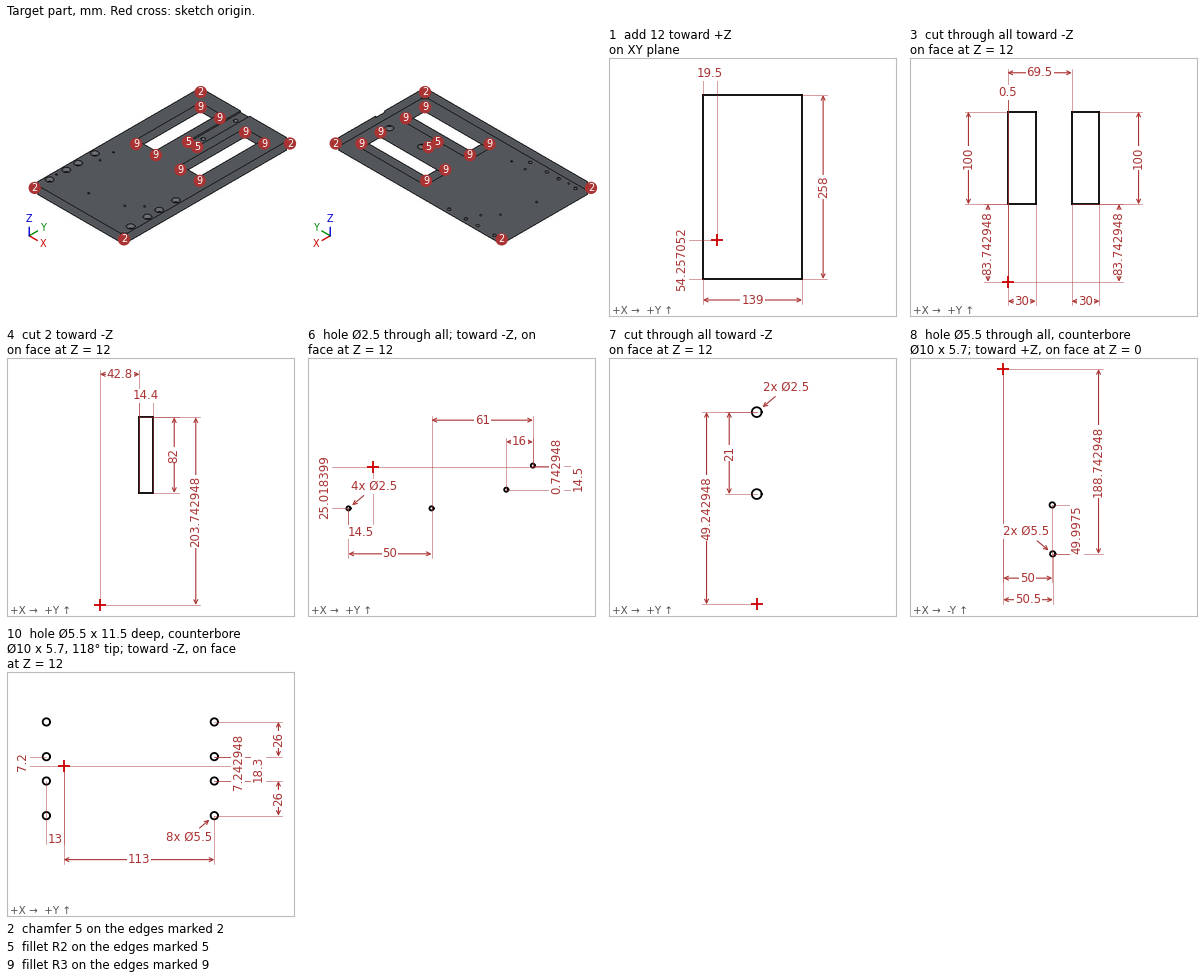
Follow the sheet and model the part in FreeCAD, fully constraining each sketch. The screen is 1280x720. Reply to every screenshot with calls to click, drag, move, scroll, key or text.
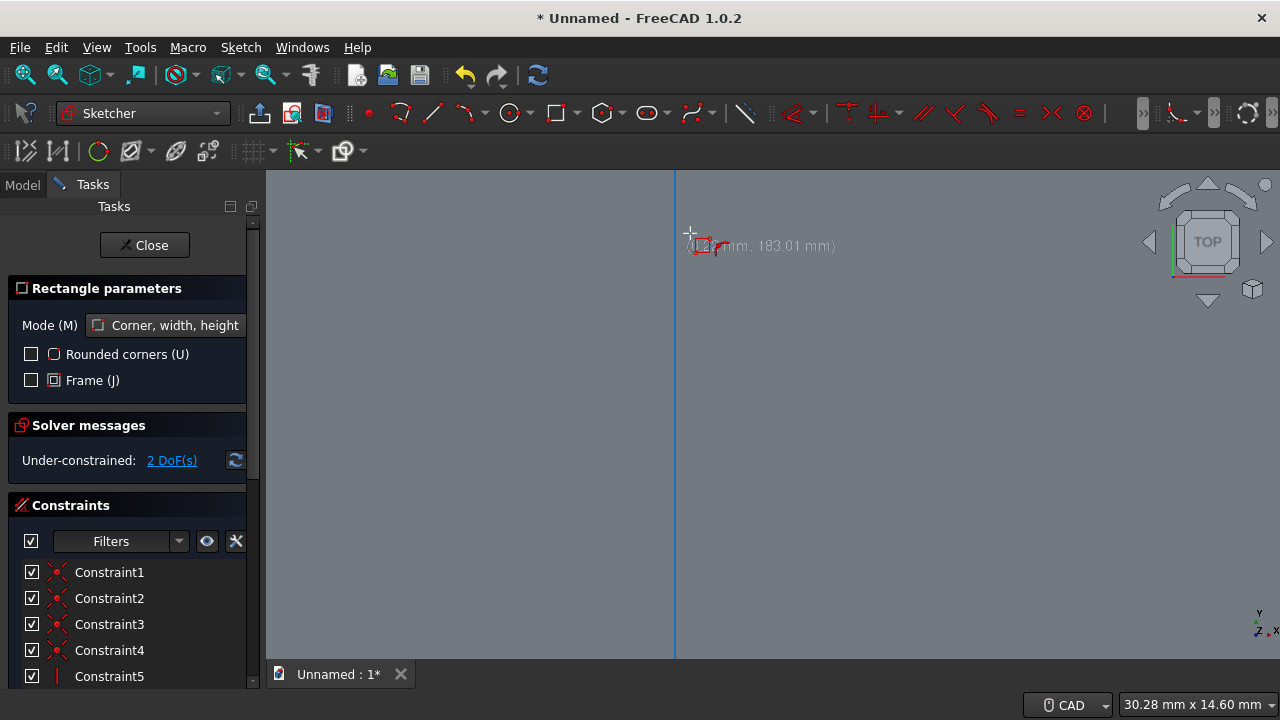
click(692, 226)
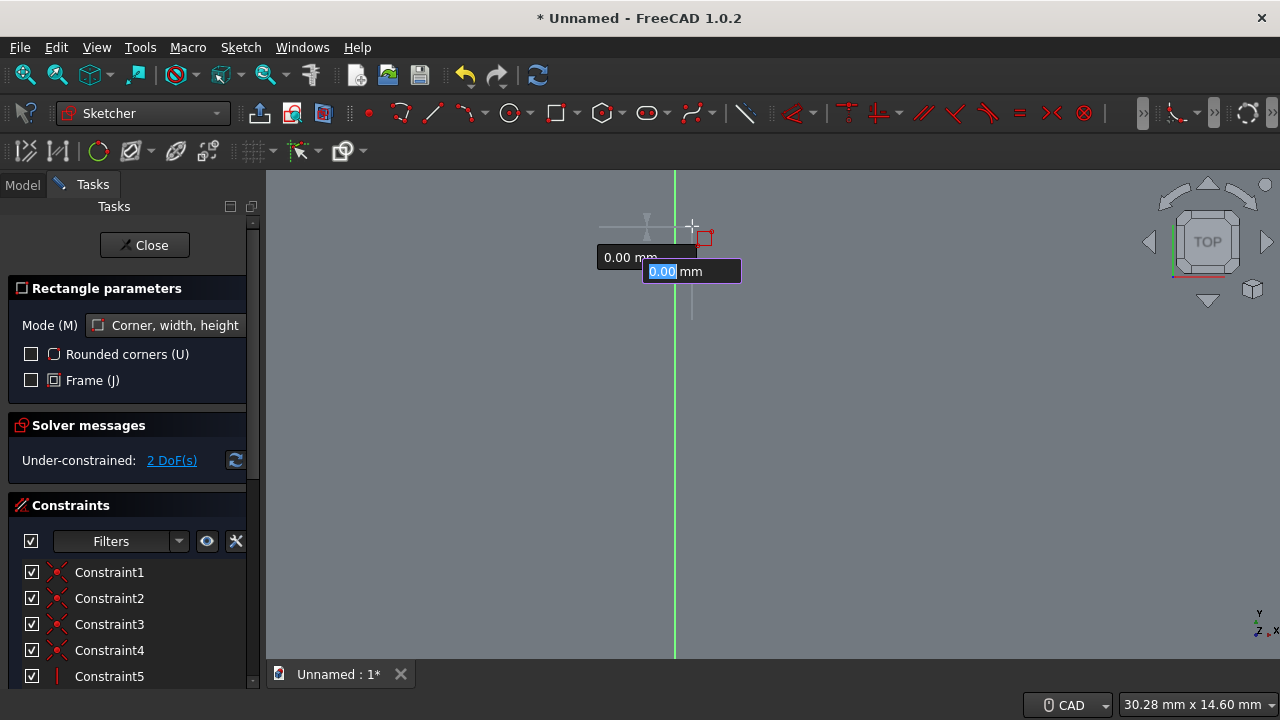
scroll(619, 263, down, 15)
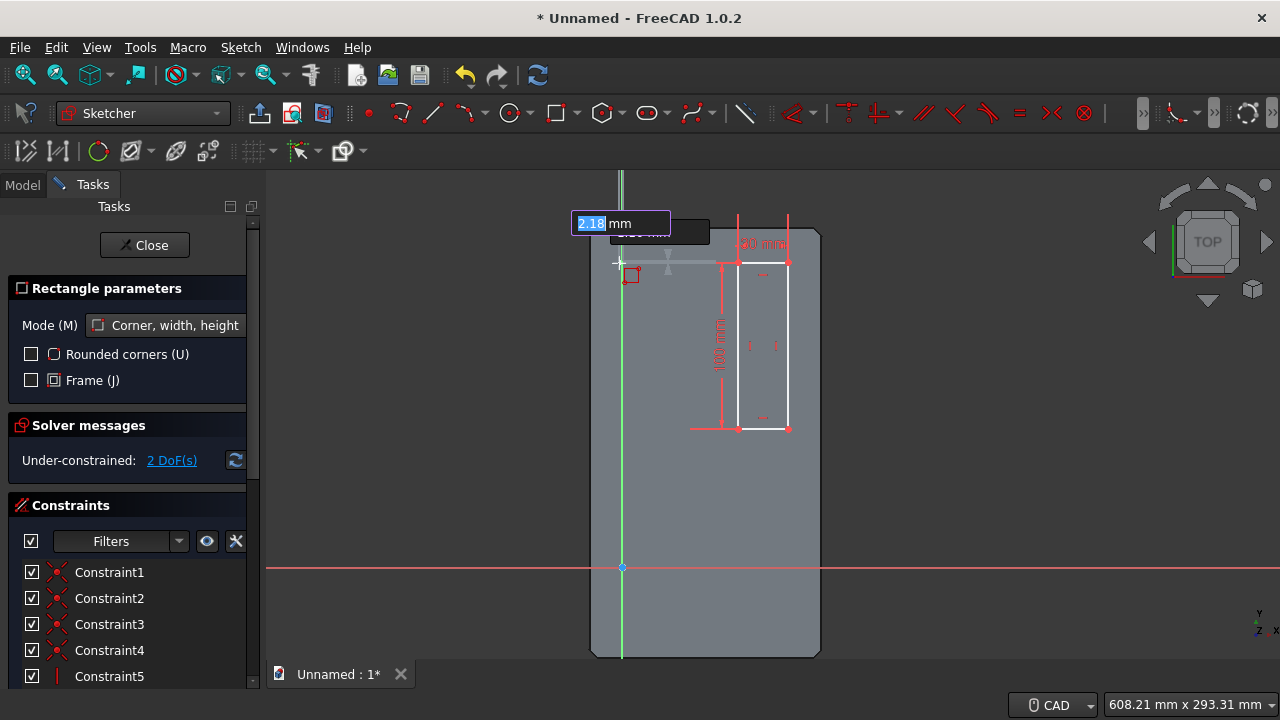
click(673, 428)
key(Escape)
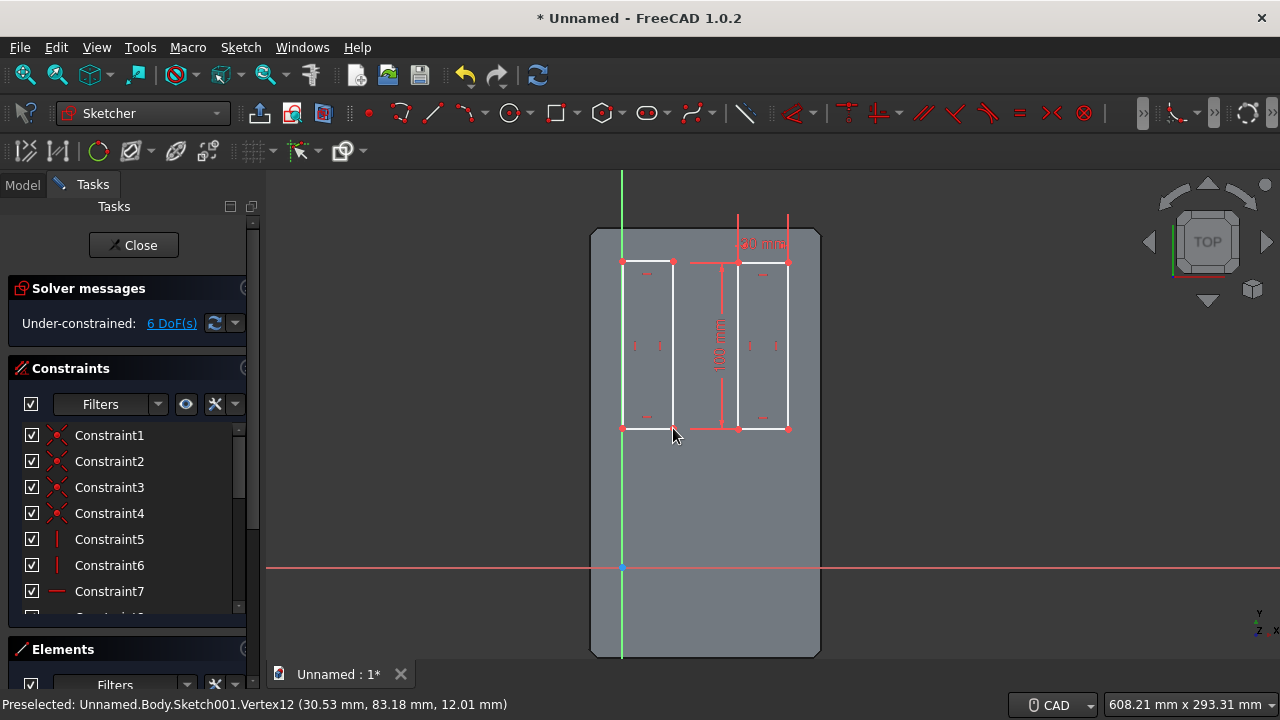
key(d)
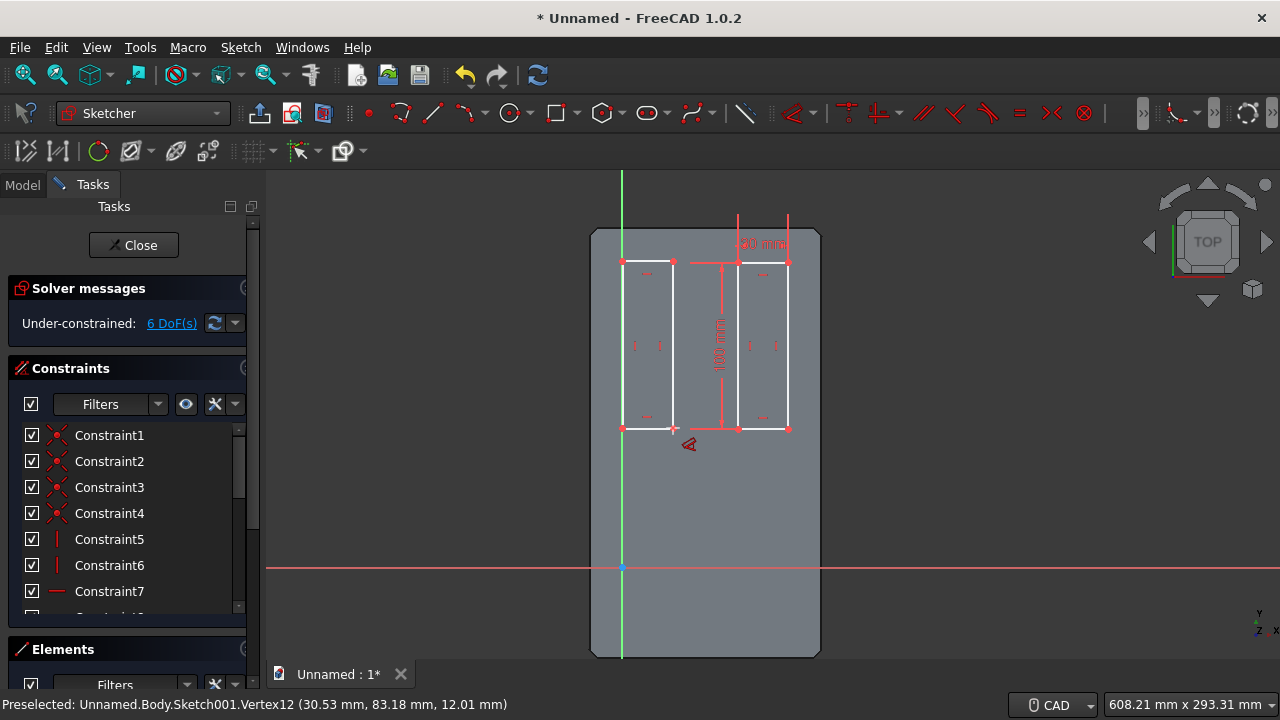
click(638, 429)
click(648, 463)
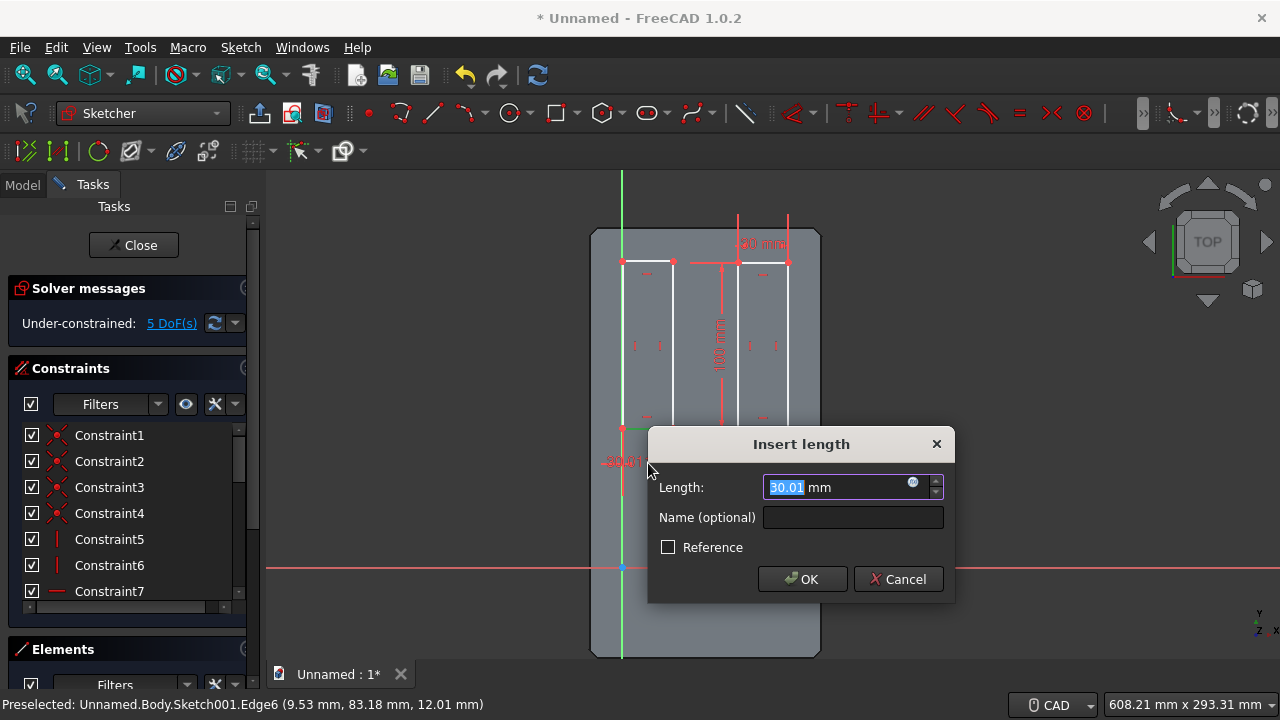
text(30)
key(Return)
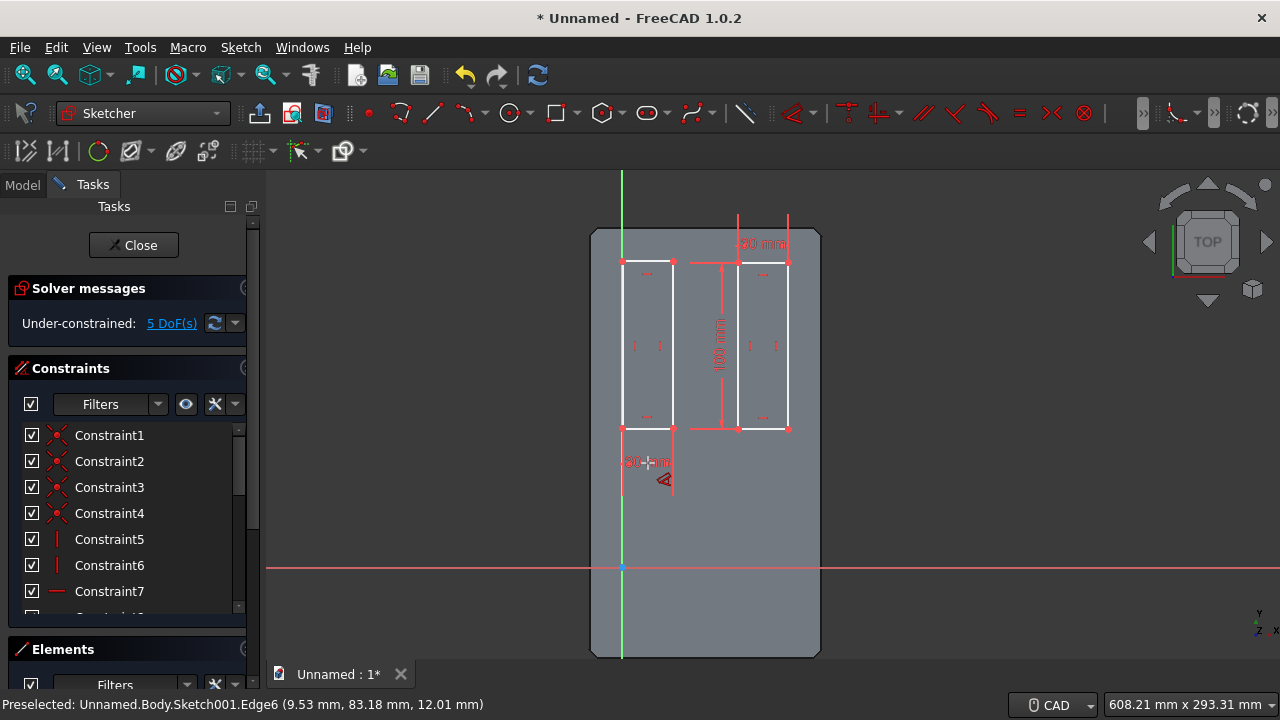
click(623, 312)
click(589, 345)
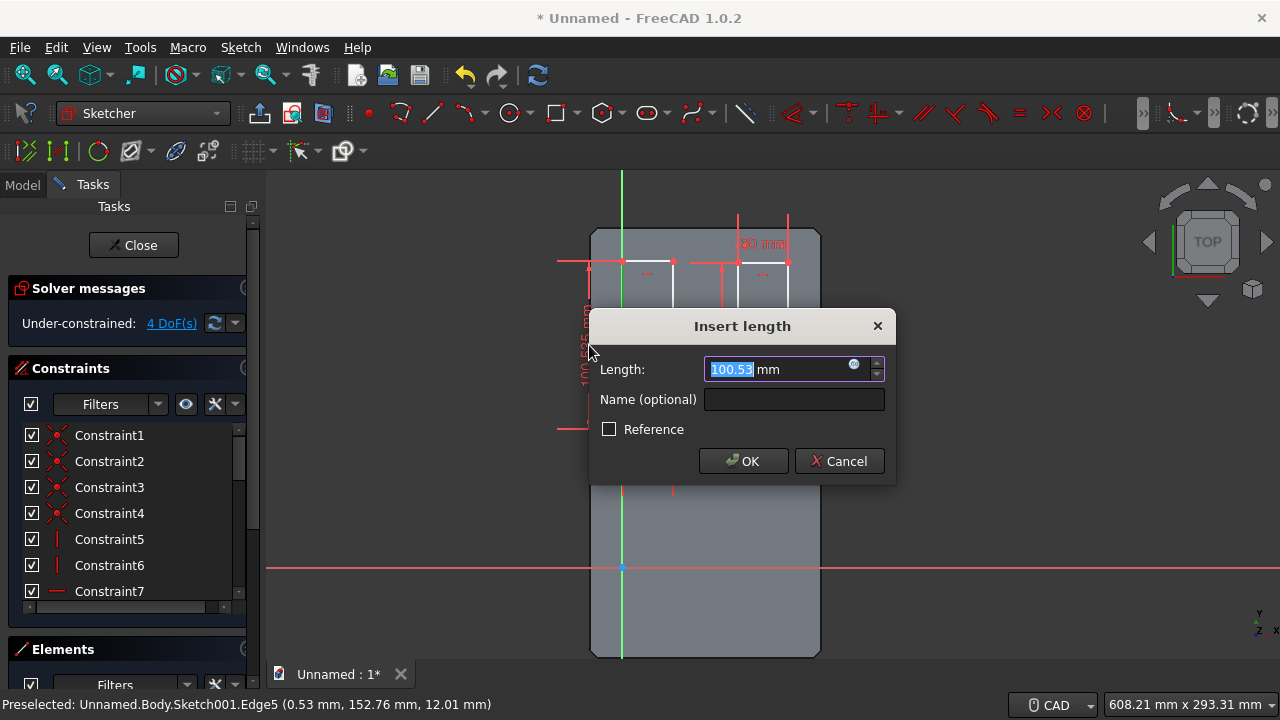
text(100)
key(Return)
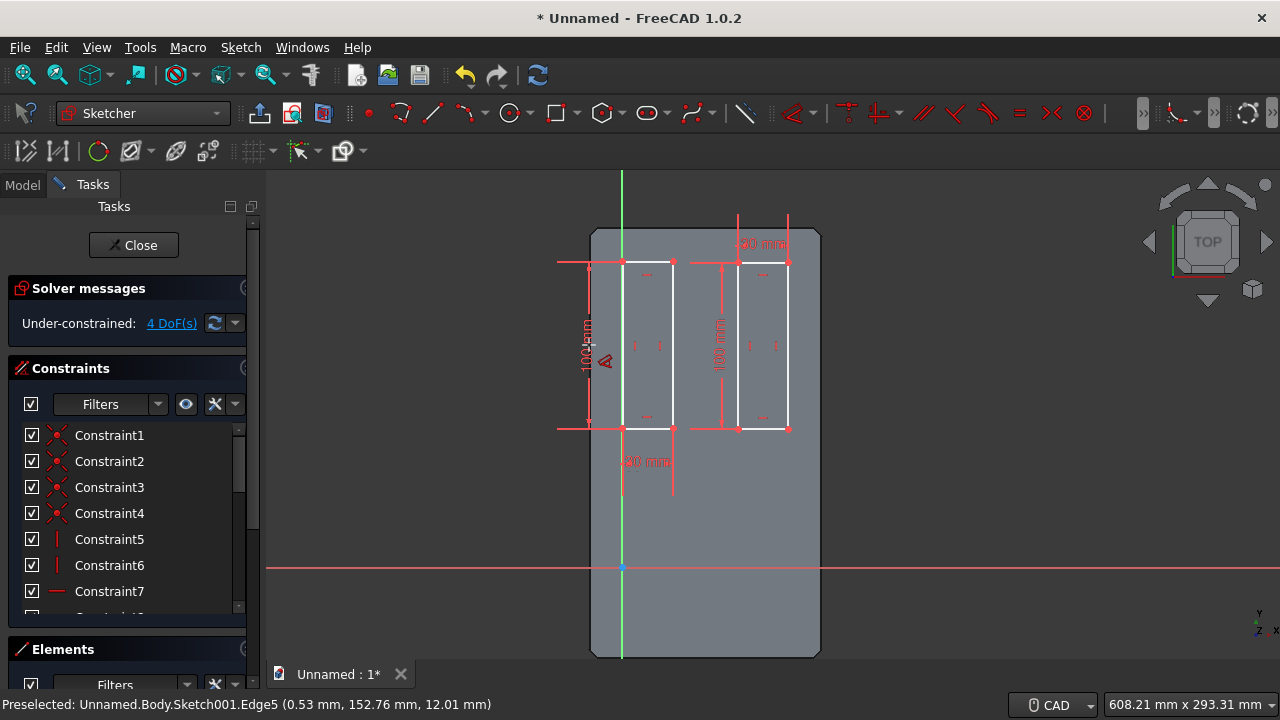
scroll(623, 262, up, 20)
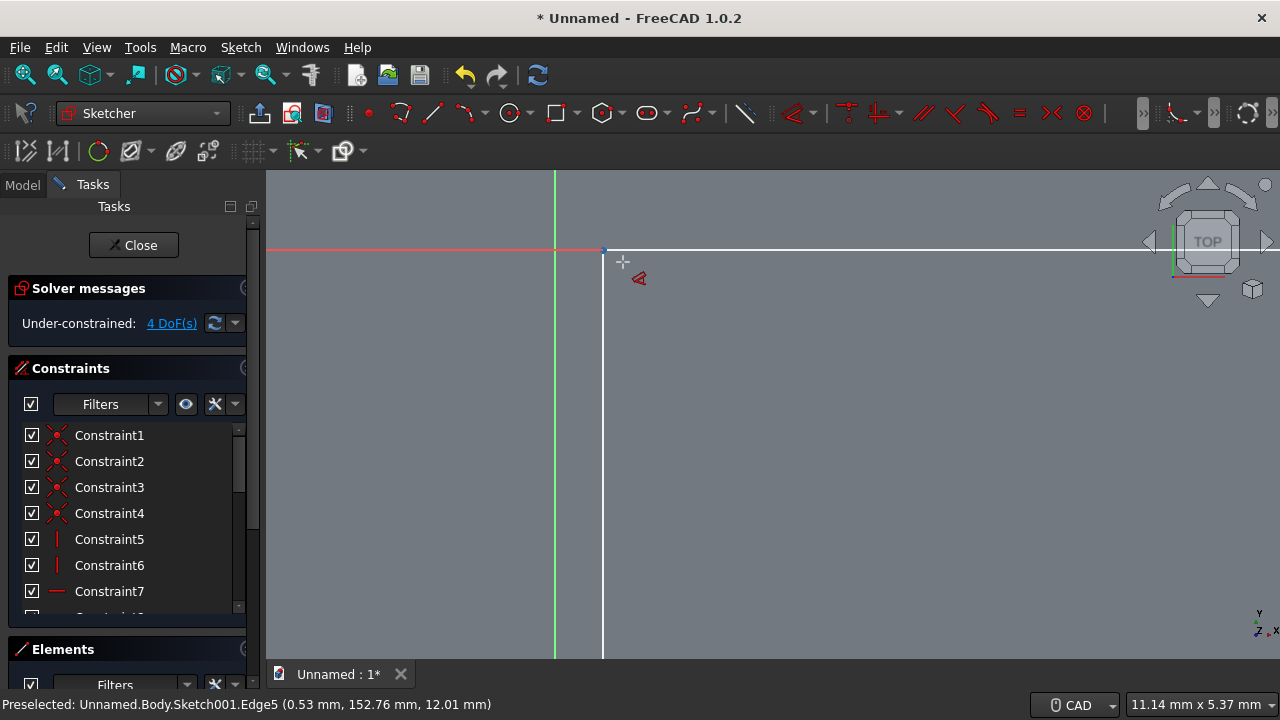
click(603, 250)
click(579, 216)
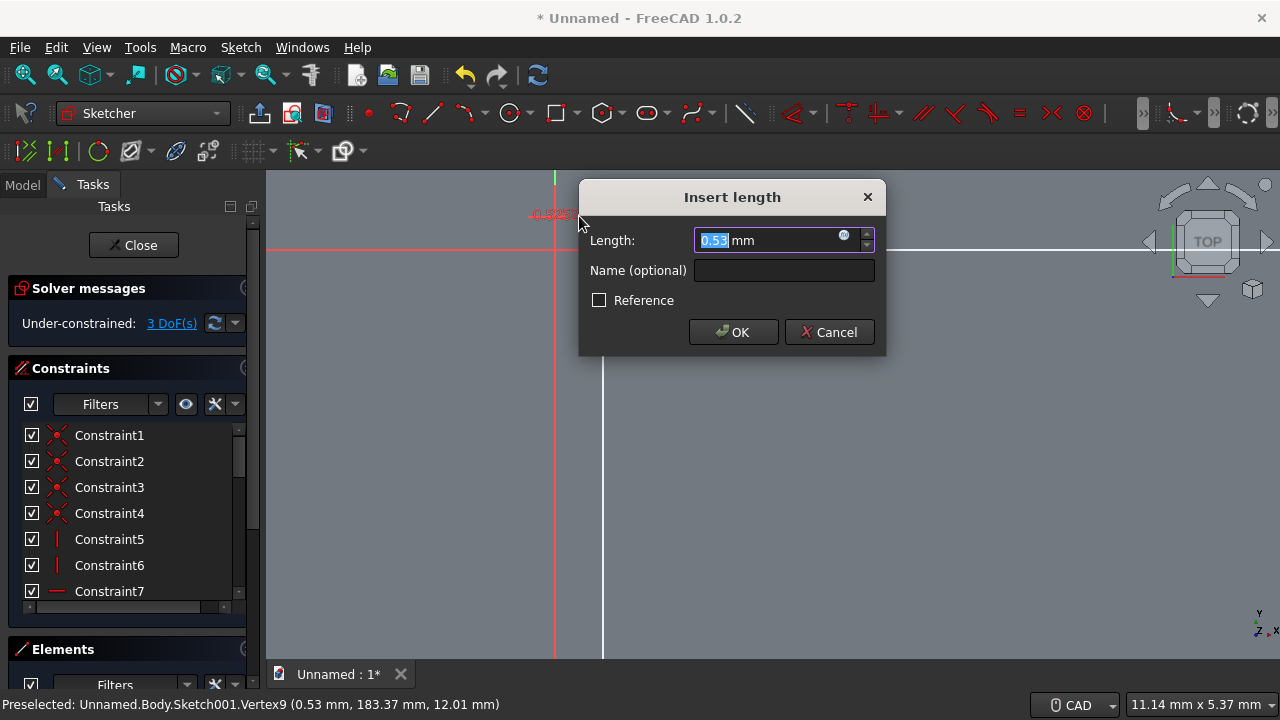
text(0.5)
key(Return)